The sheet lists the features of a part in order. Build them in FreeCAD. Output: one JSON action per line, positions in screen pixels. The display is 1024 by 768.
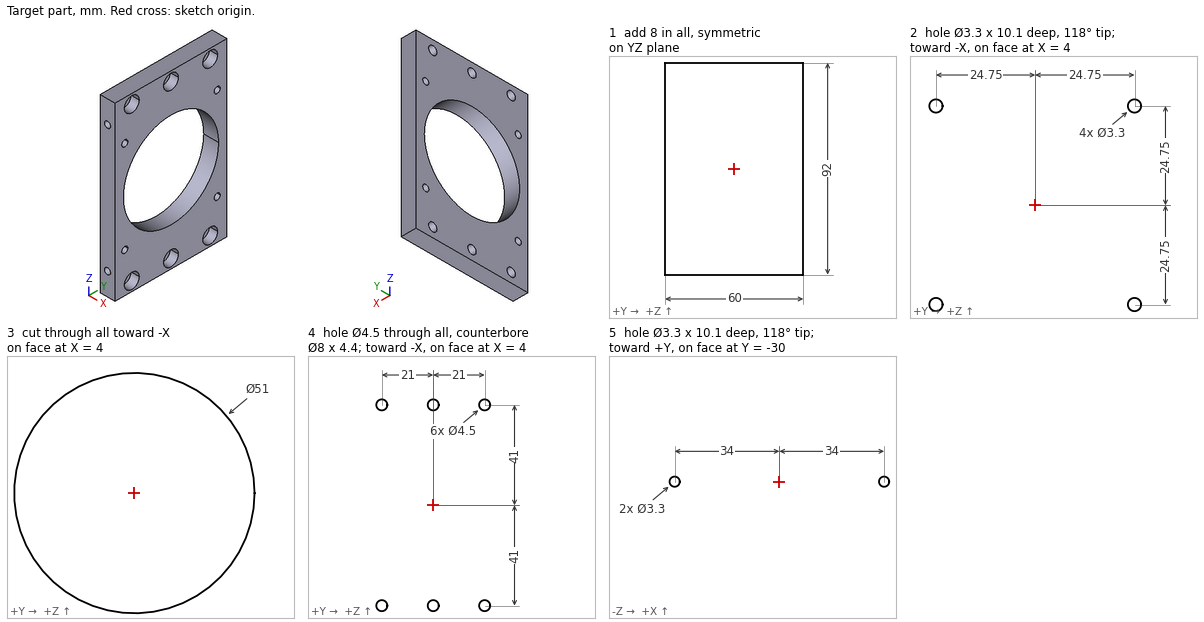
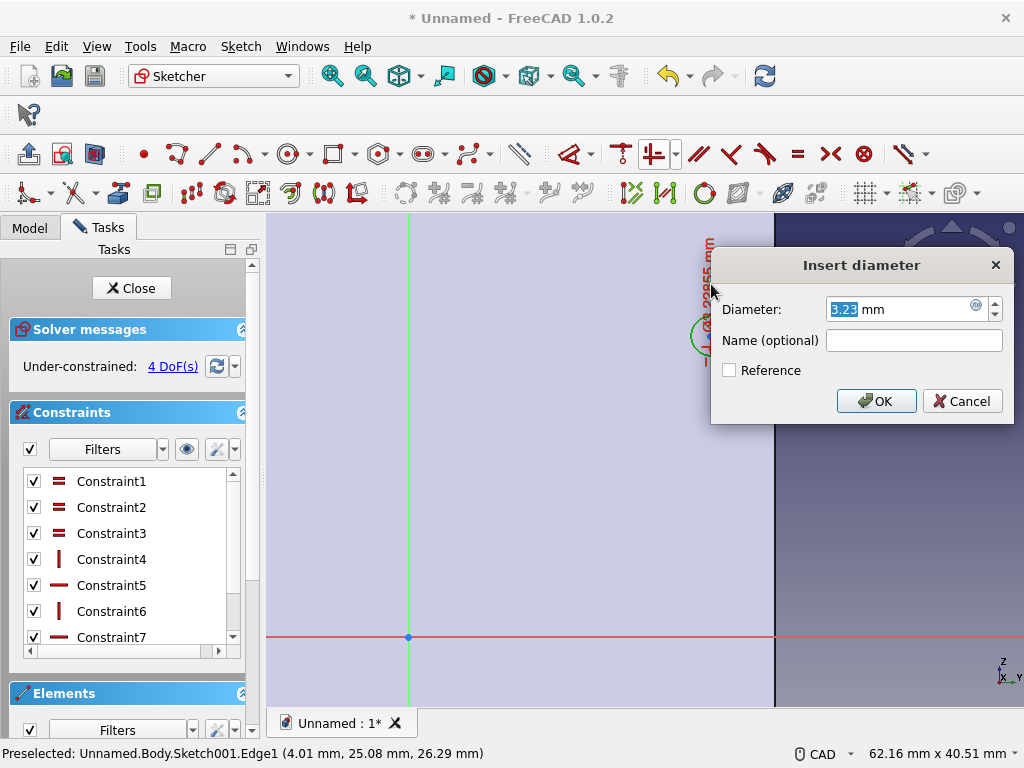
{"action": "type", "text": "3.3"}
{"action": "key", "text": "Return"}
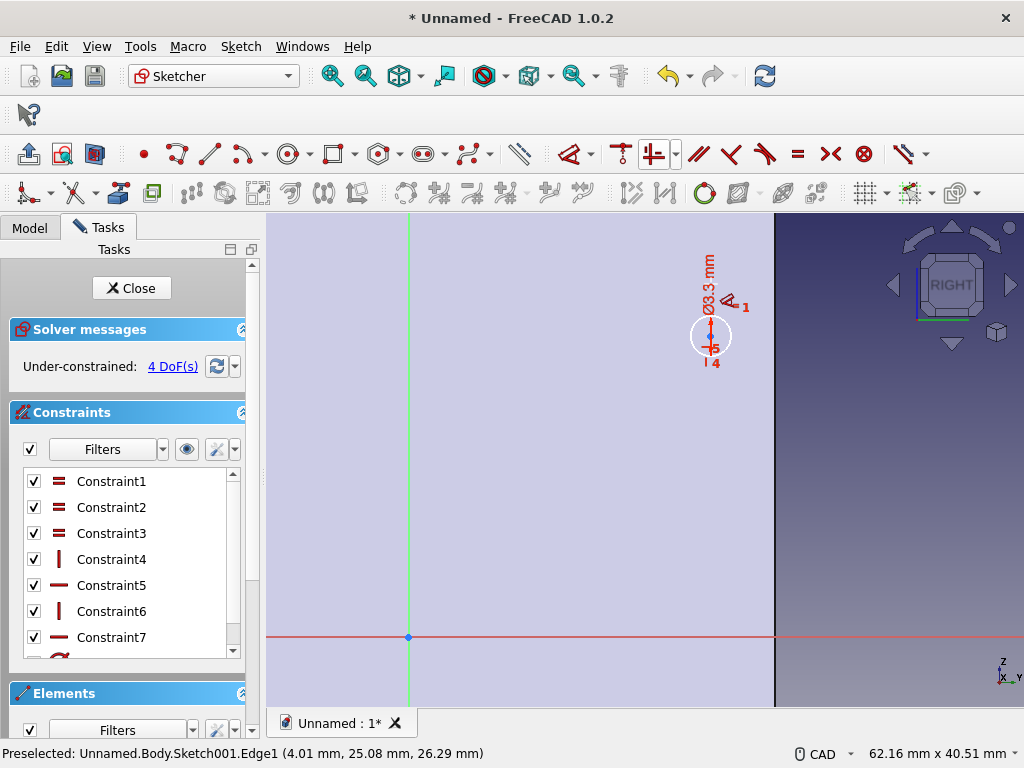
{"action": "left_click", "coordinate": [711, 336]}
{"action": "left_click", "coordinate": [560, 302]}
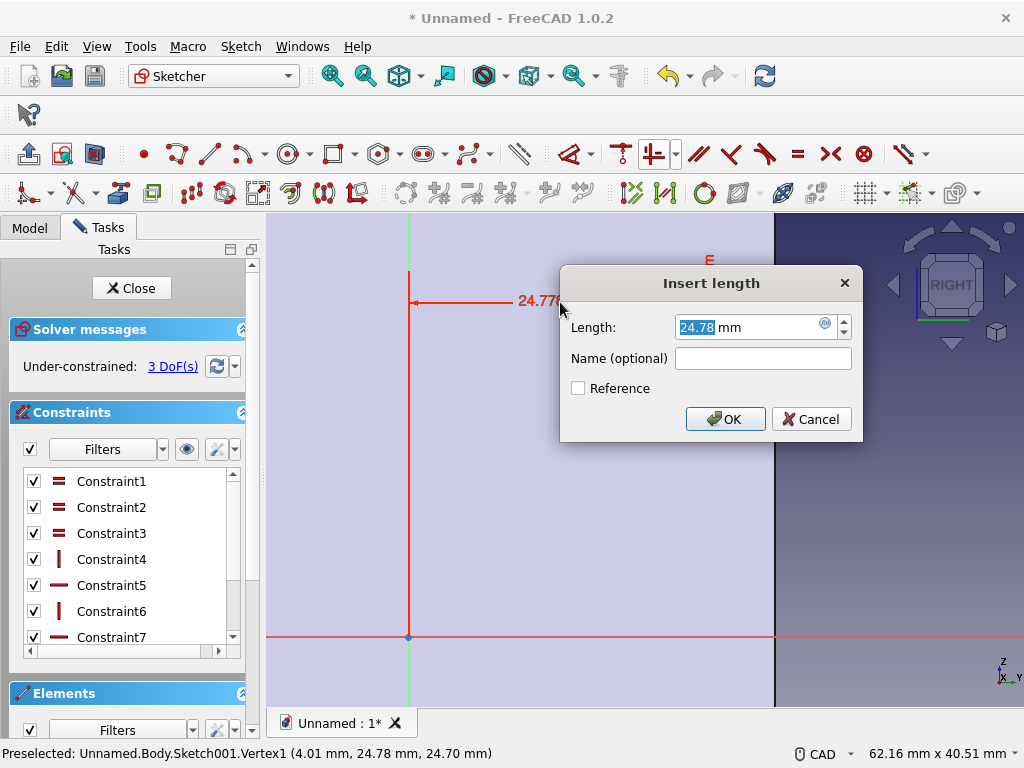
{"action": "type", "text": "24.75"}
{"action": "key", "text": "Return"}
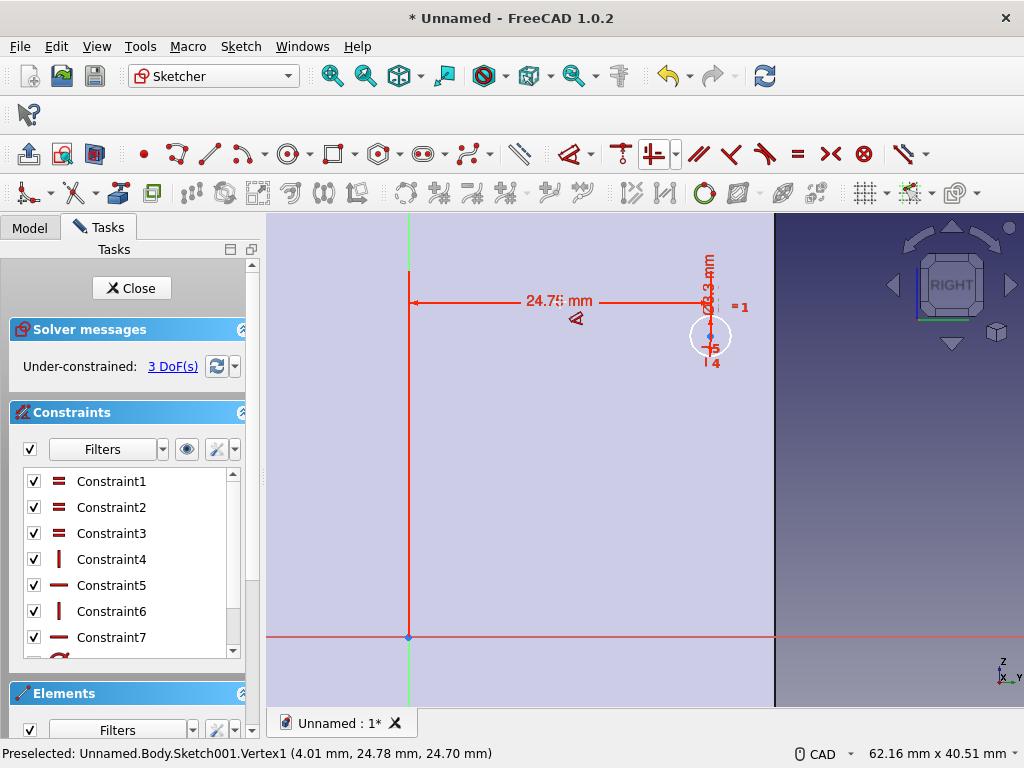
{"action": "left_click", "coordinate": [711, 336]}
{"action": "left_click", "coordinate": [745, 487]}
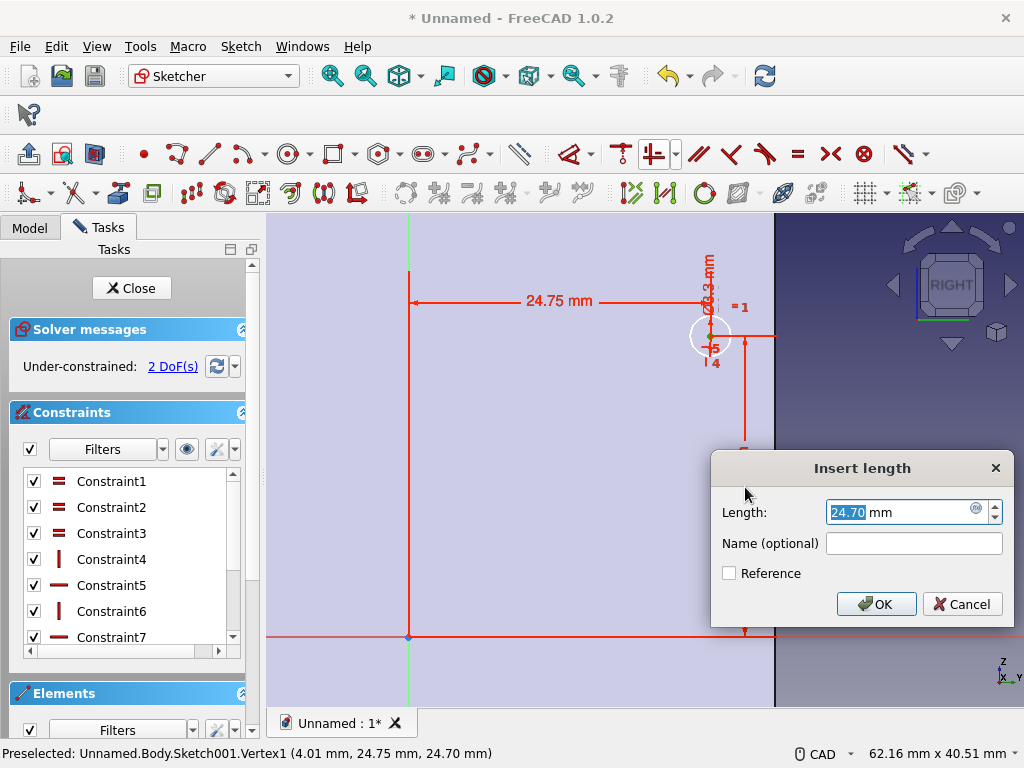
{"action": "type", "text": "24.75"}
{"action": "key", "text": "Return"}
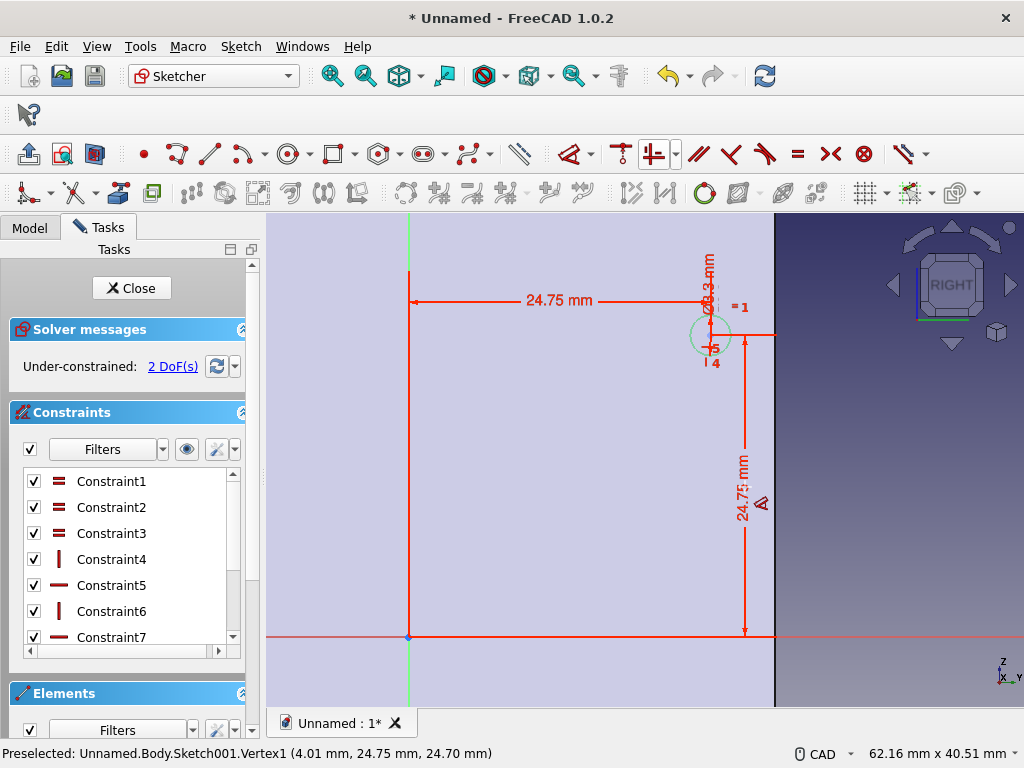
{"action": "scroll", "coordinate": [713, 315], "scroll_direction": "down", "scroll_amount": 4}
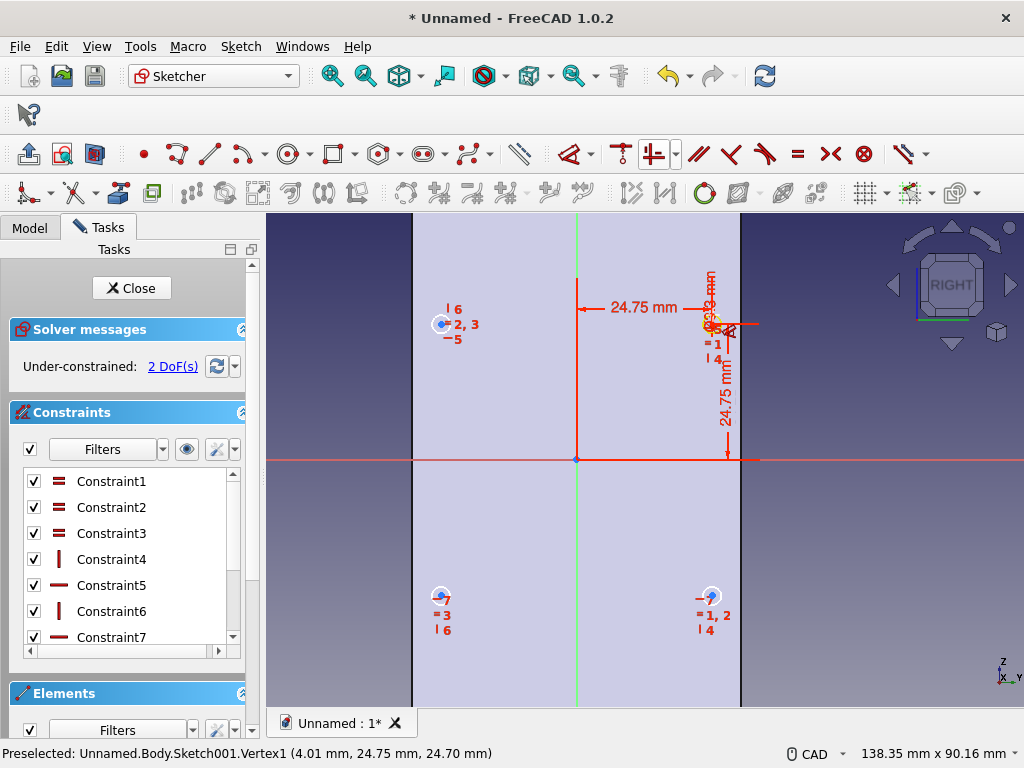
{"action": "left_click", "coordinate": [712, 596]}
{"action": "left_click", "coordinate": [746, 528]}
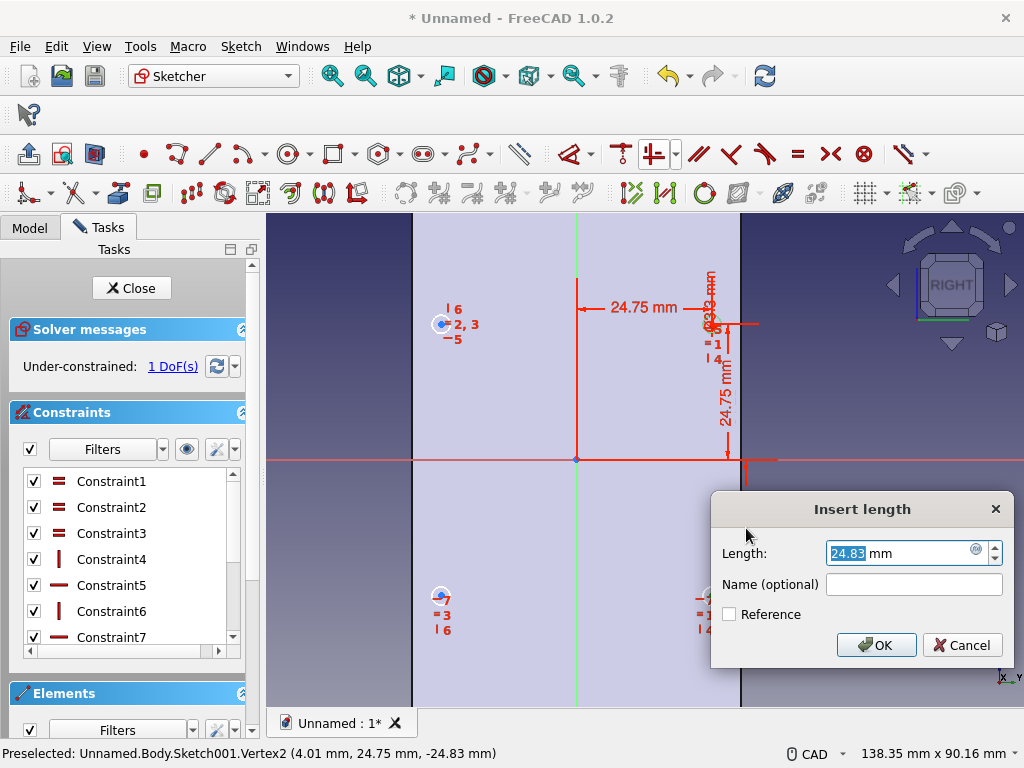
{"action": "type", "text": "24.75"}
{"action": "key", "text": "Return"}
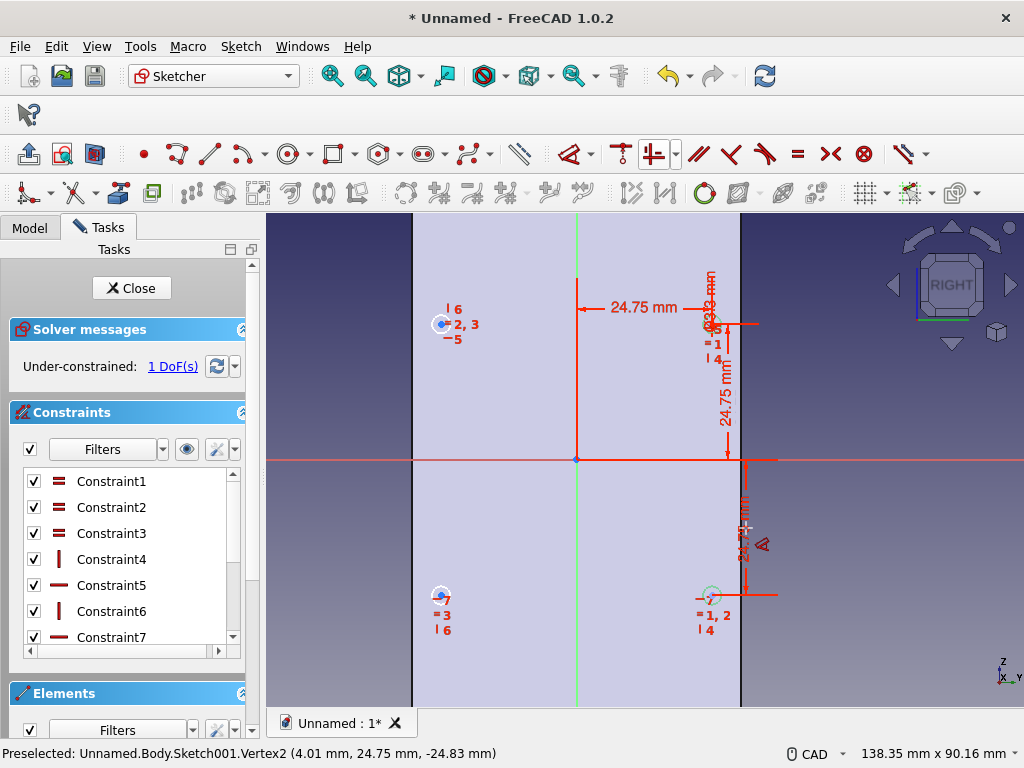
{"action": "left_click", "coordinate": [441, 324]}
{"action": "left_click", "coordinate": [509, 290]}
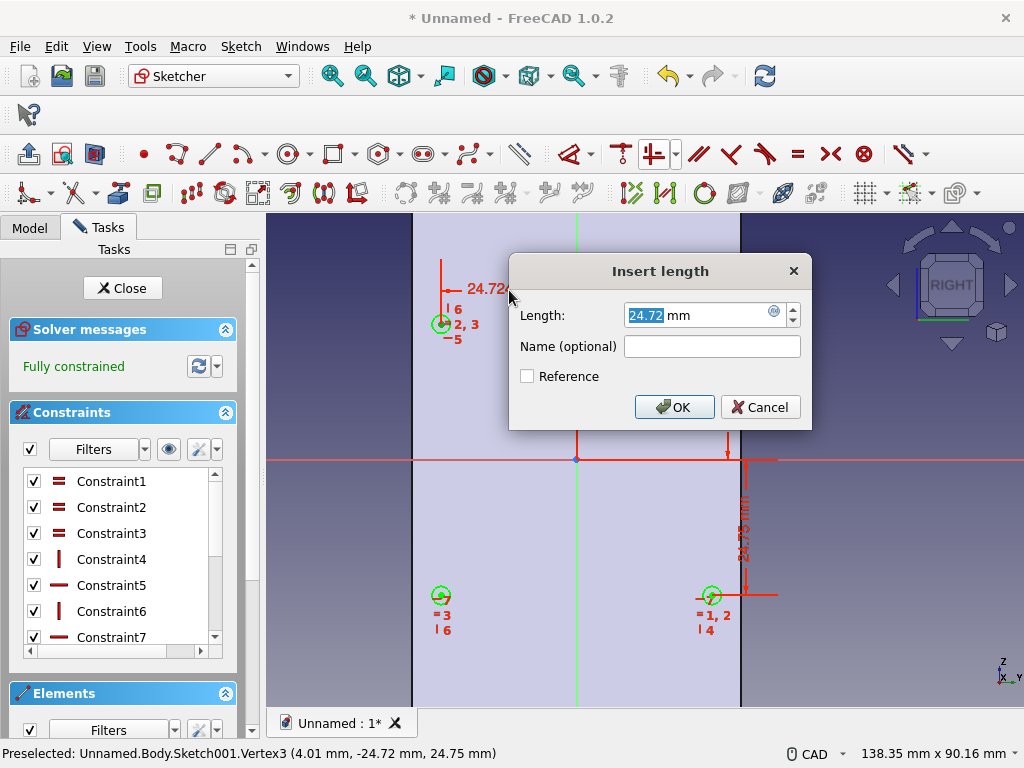
{"action": "type", "text": "24.75"}
{"action": "key", "text": "Return"}
{"action": "key", "text": "Escape"}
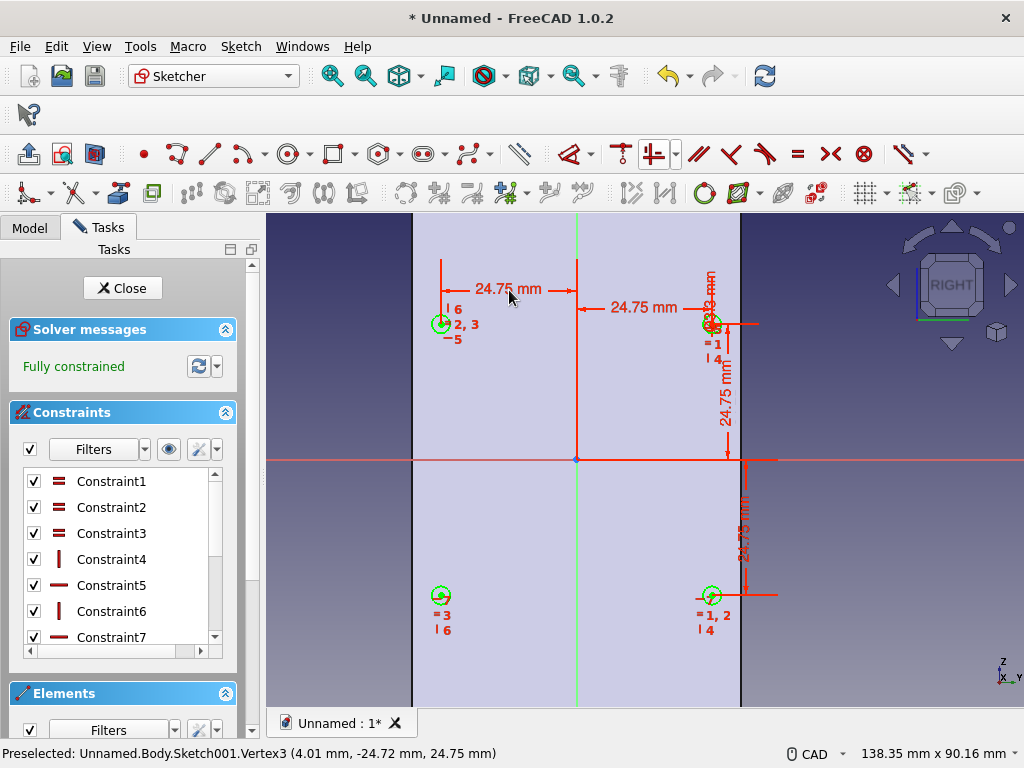
{"action": "left_click", "coordinate": [123, 288]}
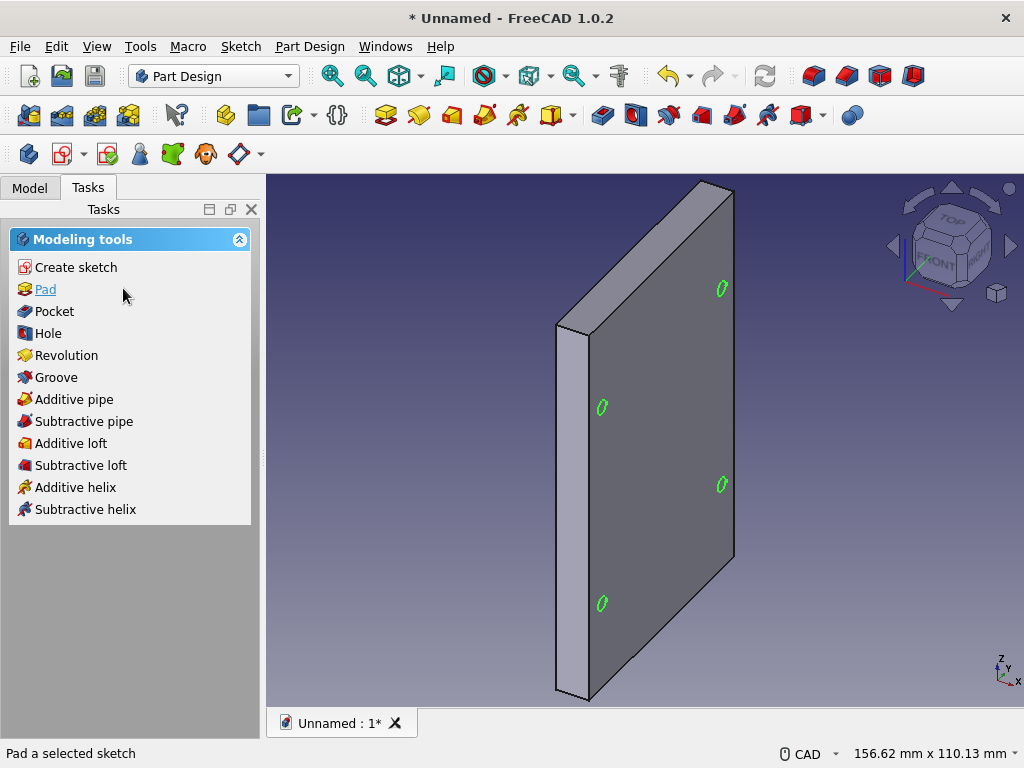
{"action": "left_click", "coordinate": [636, 116]}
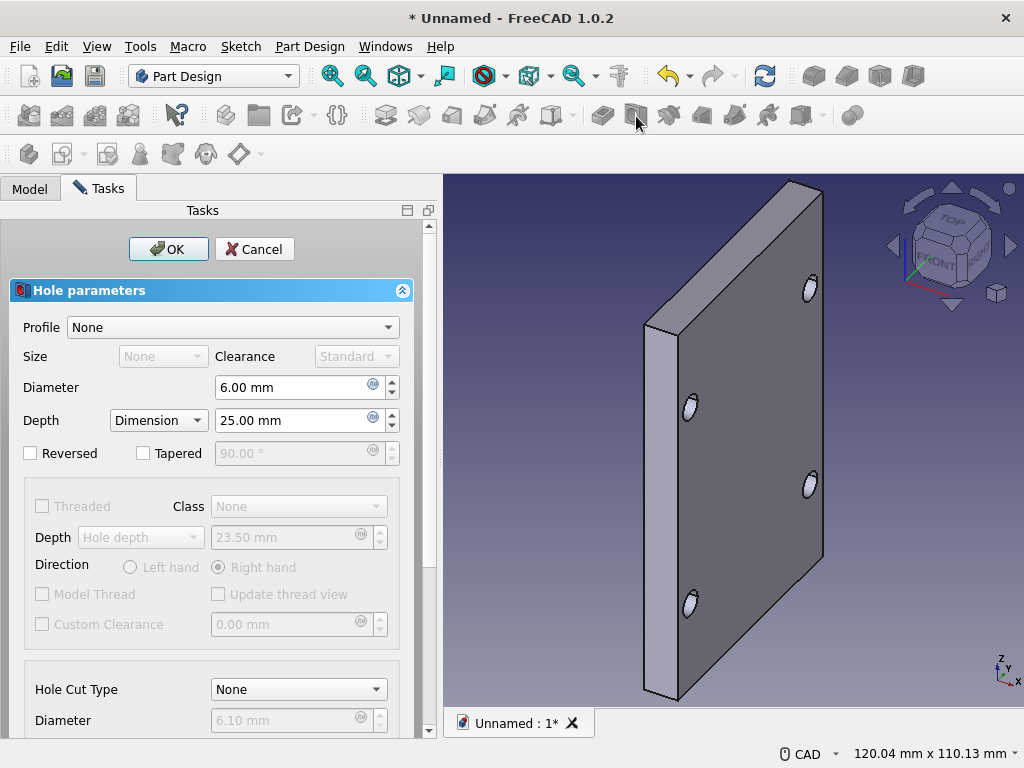
{"action": "triple_click", "coordinate": [300, 388]}